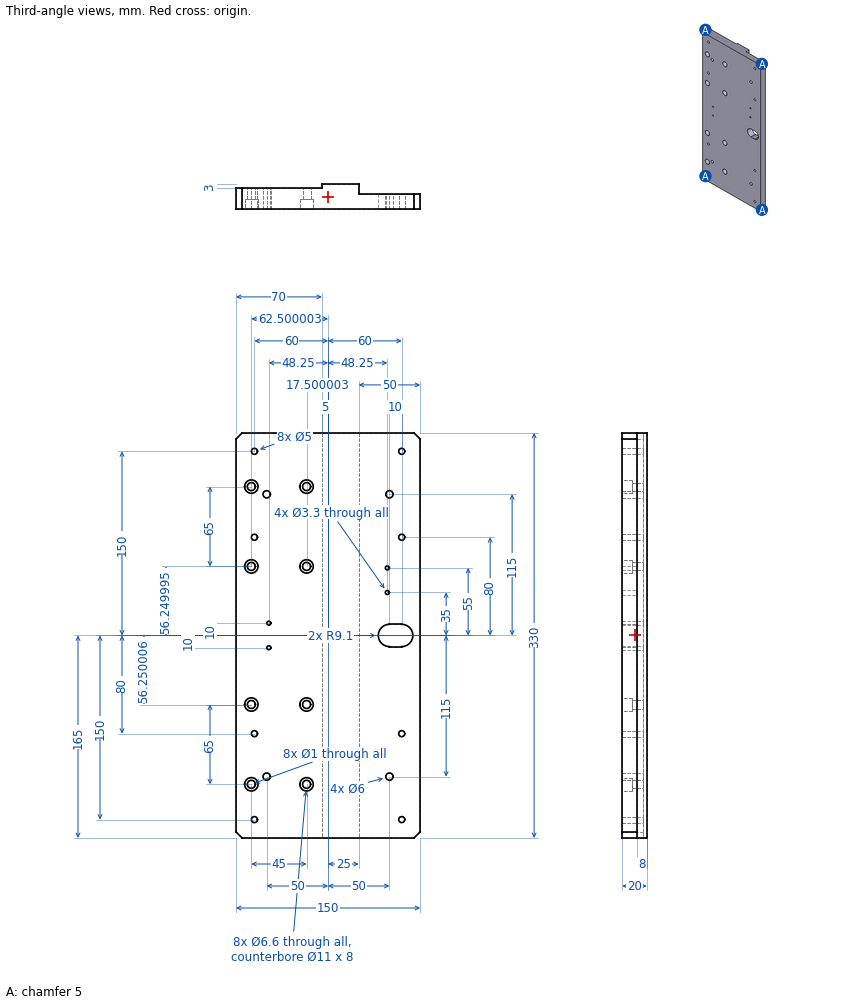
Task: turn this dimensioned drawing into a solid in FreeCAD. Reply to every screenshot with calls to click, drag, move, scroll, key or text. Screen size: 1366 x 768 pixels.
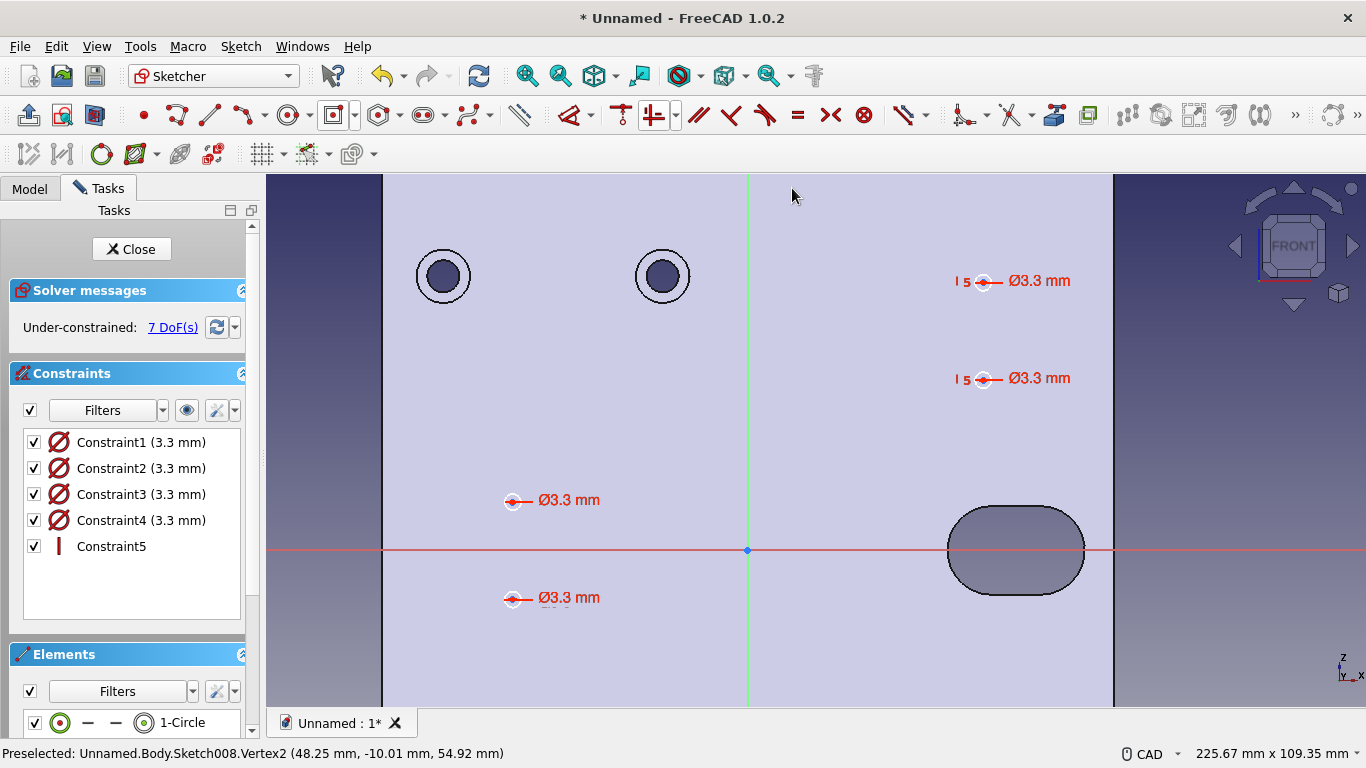
click(513, 502)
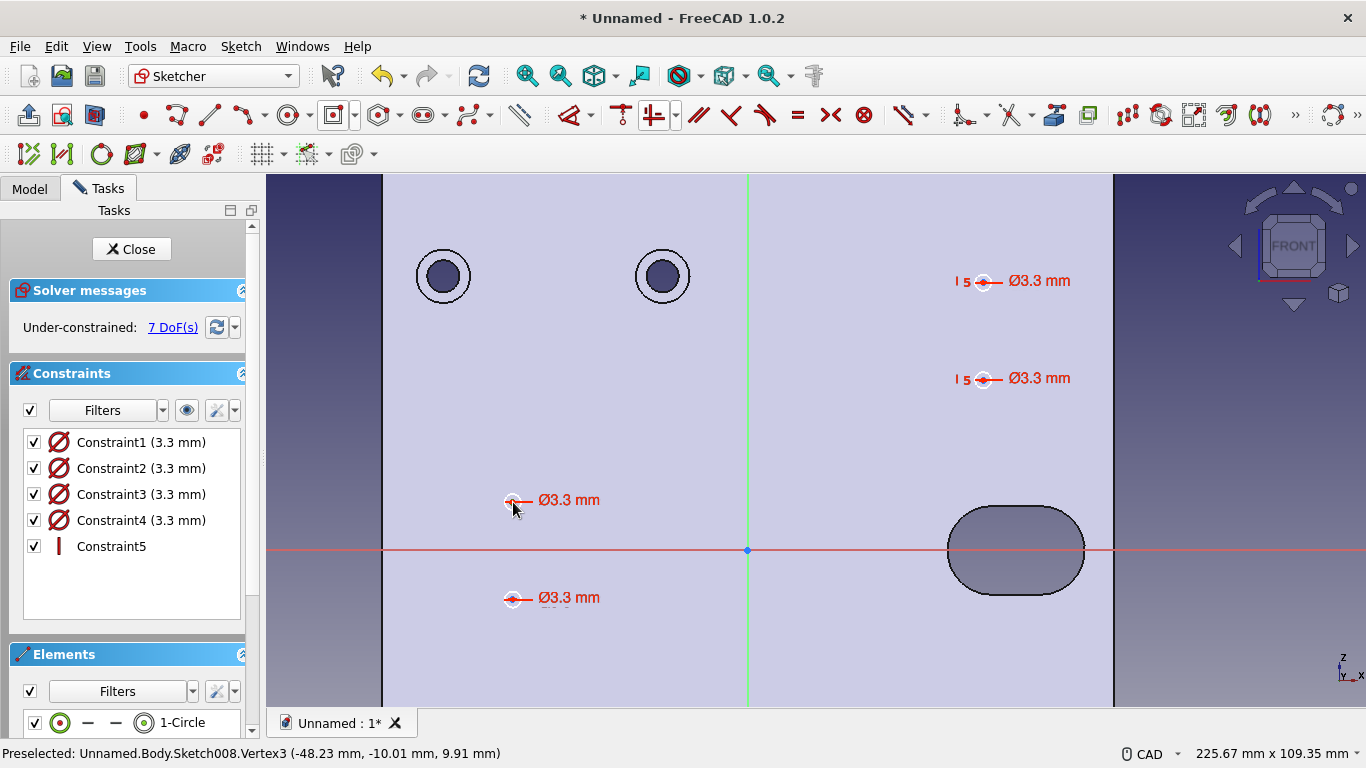
click(513, 600)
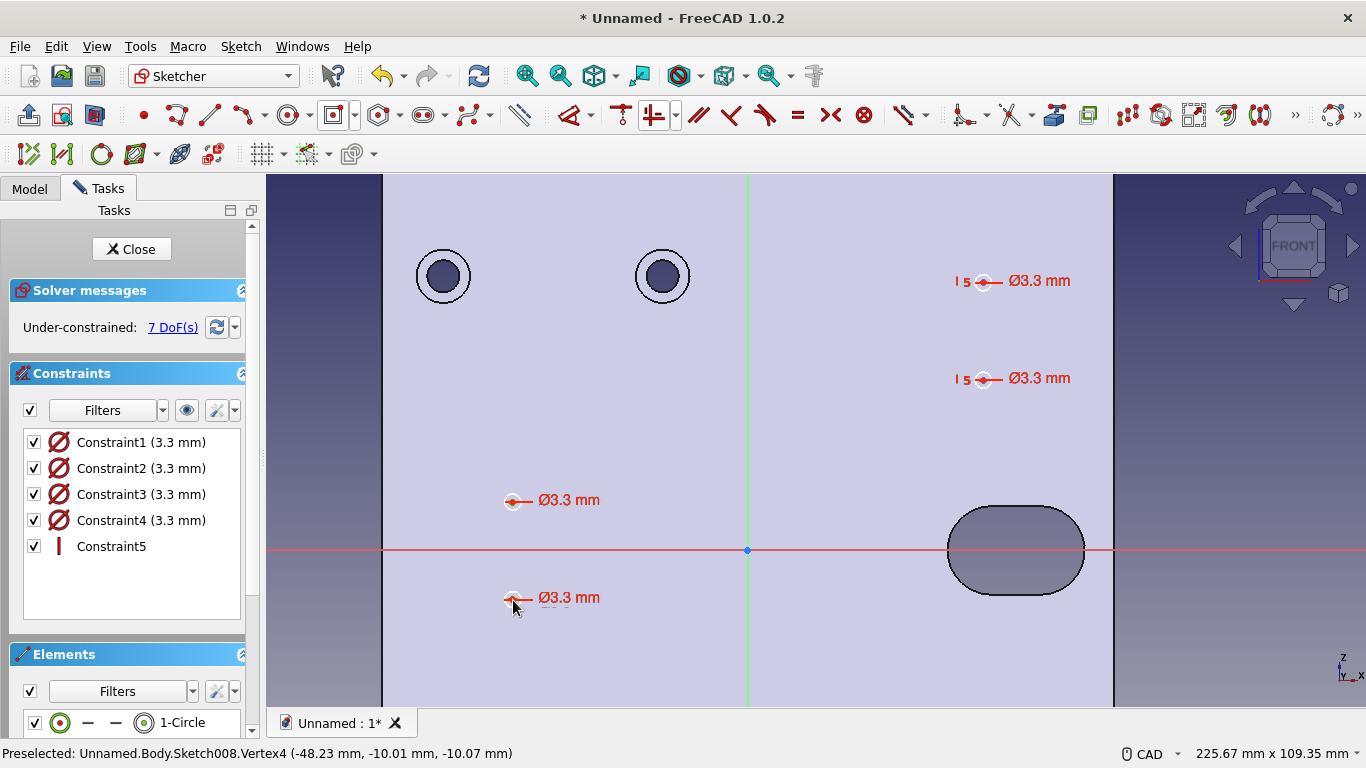
click(676, 116)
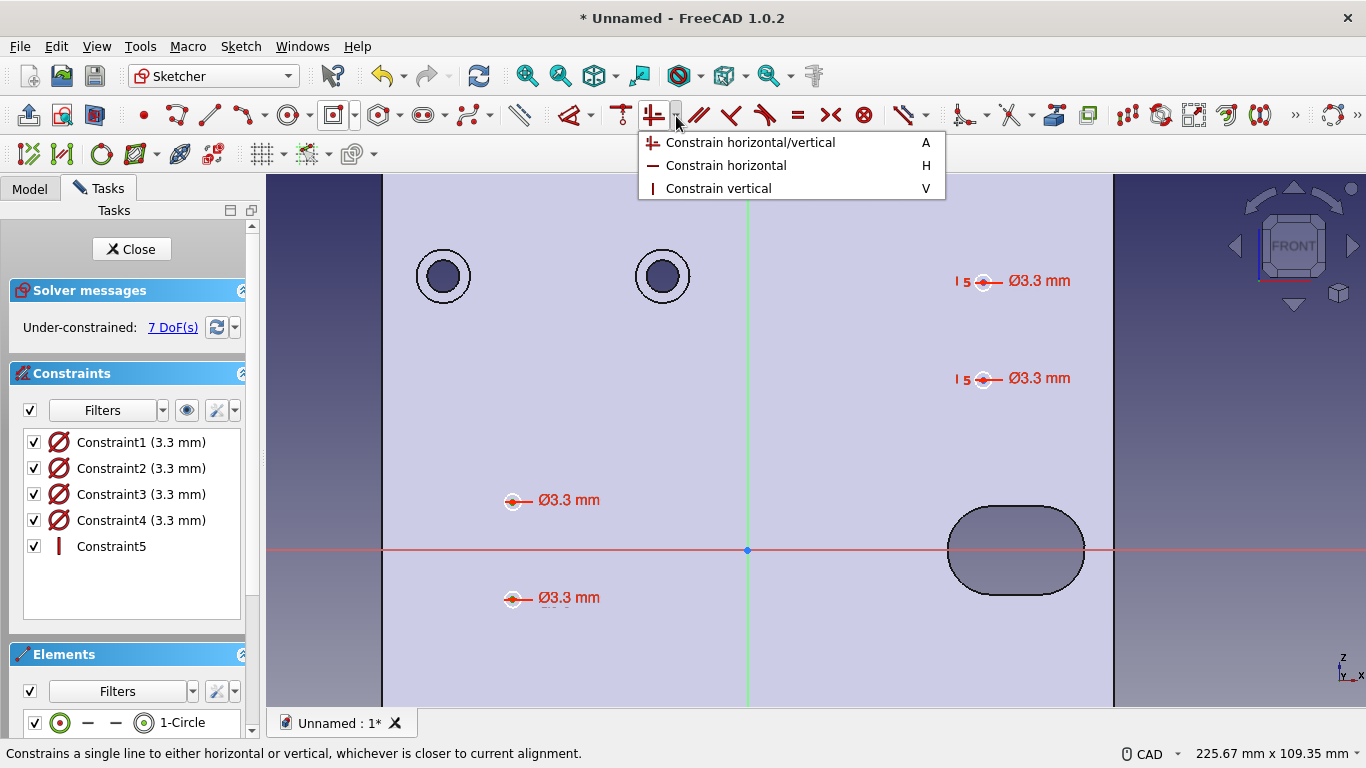
click(792, 188)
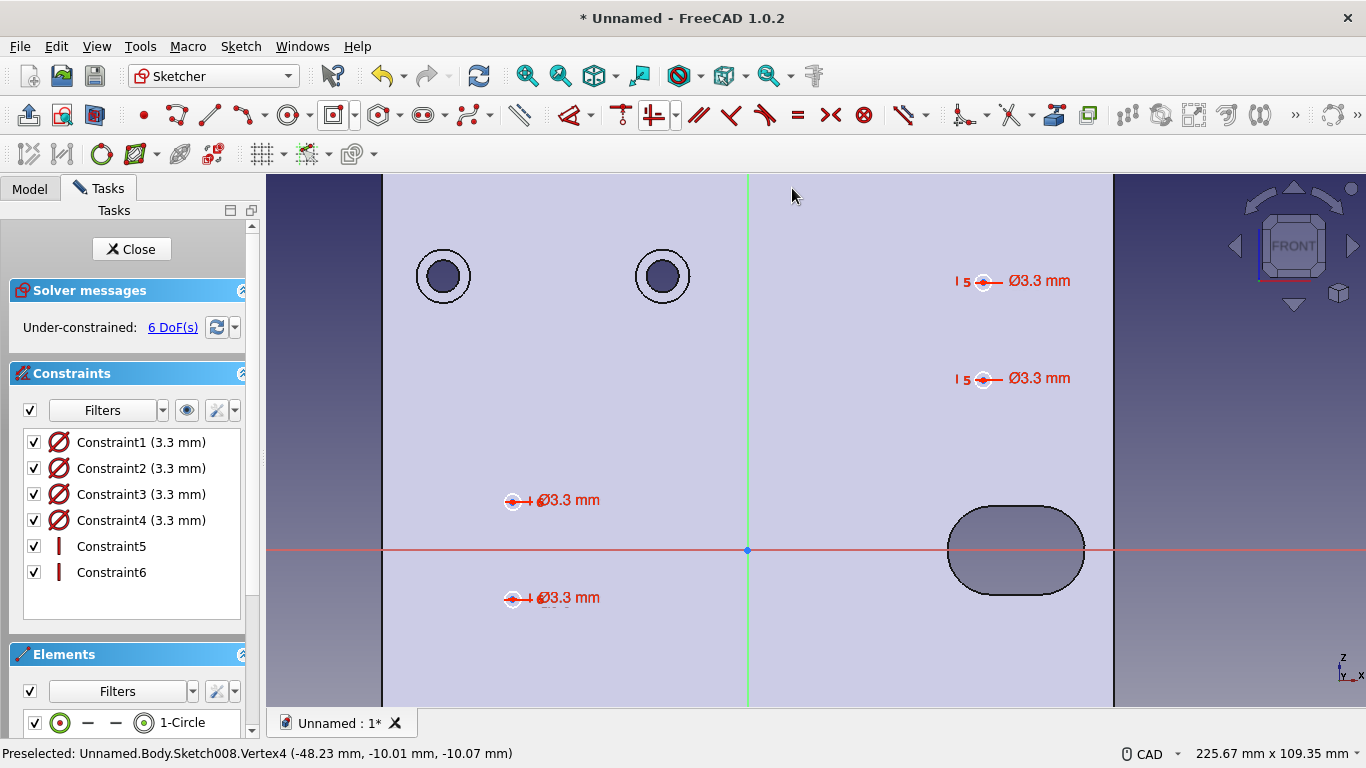
click(568, 116)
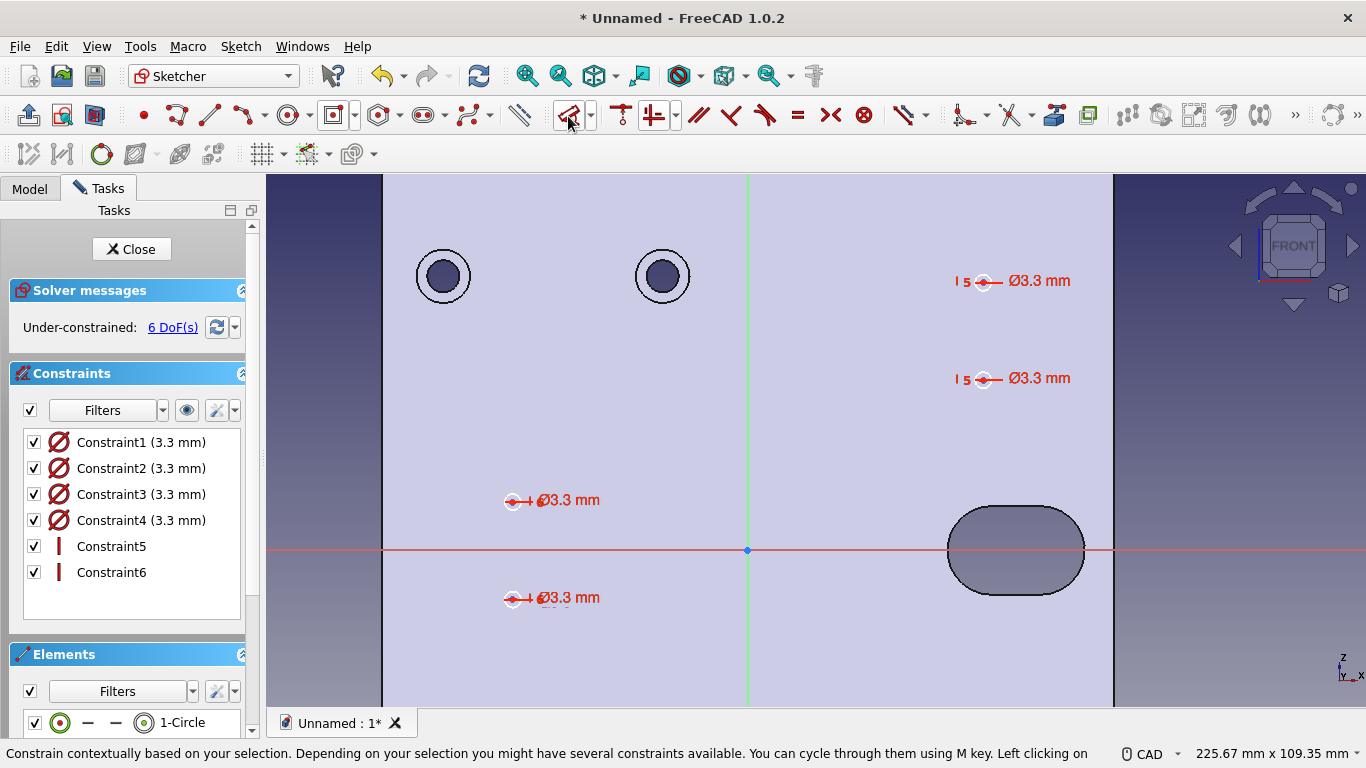
click(983, 380)
click(1017, 465)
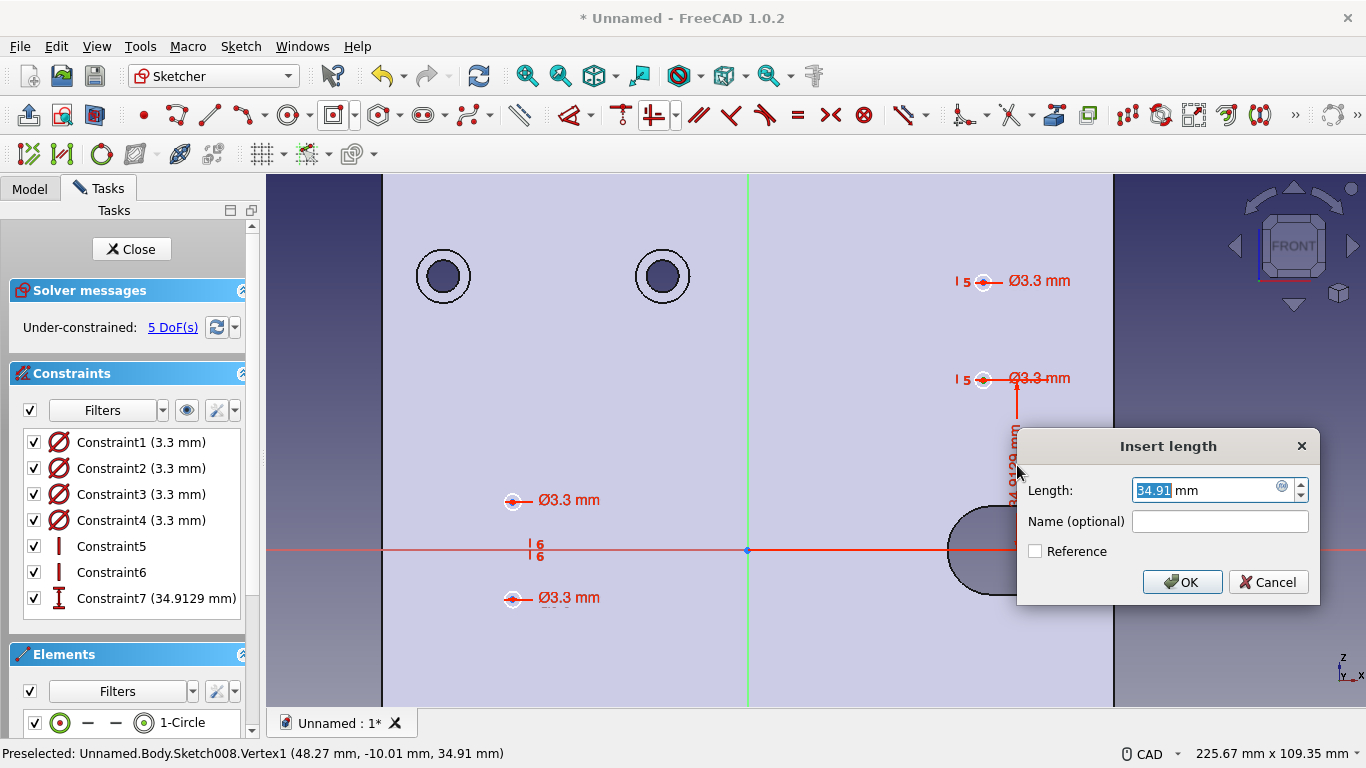
text(35)
key(Return)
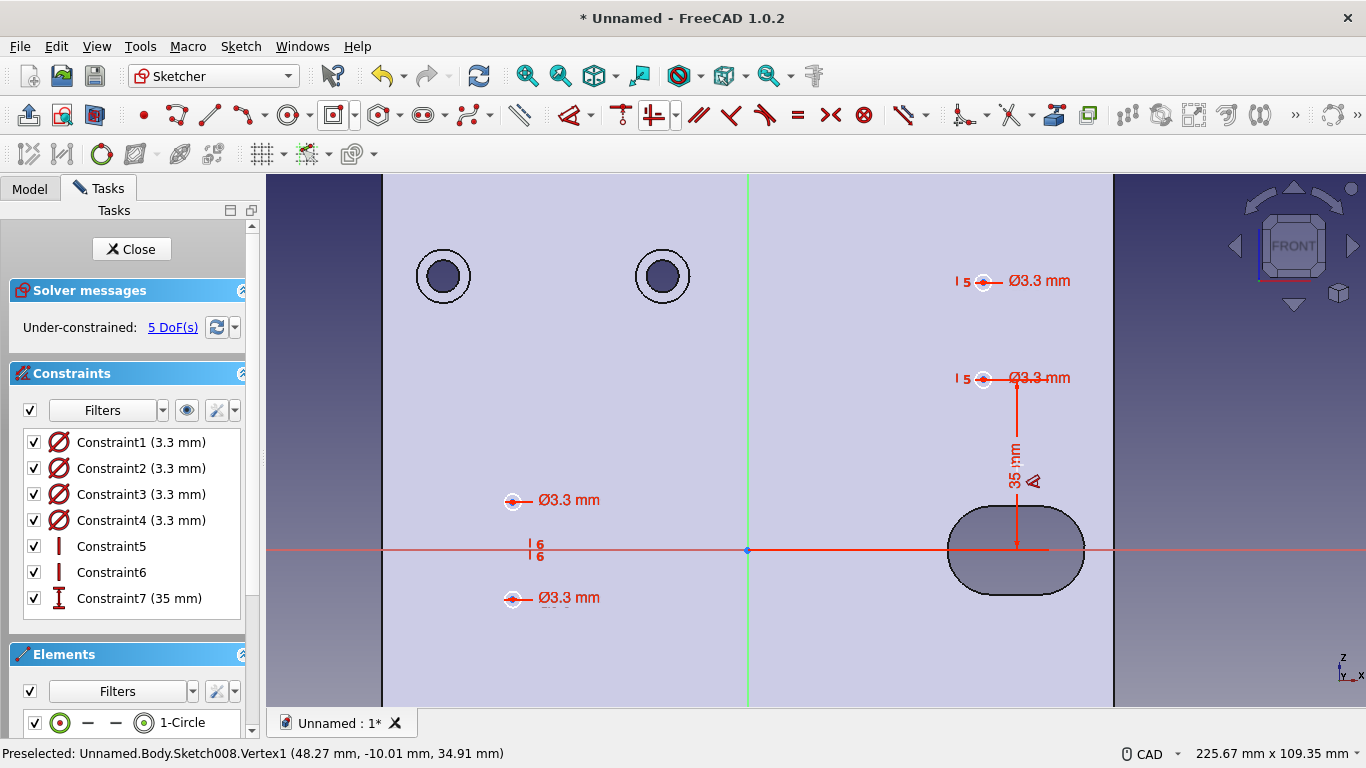
click(983, 283)
click(1017, 417)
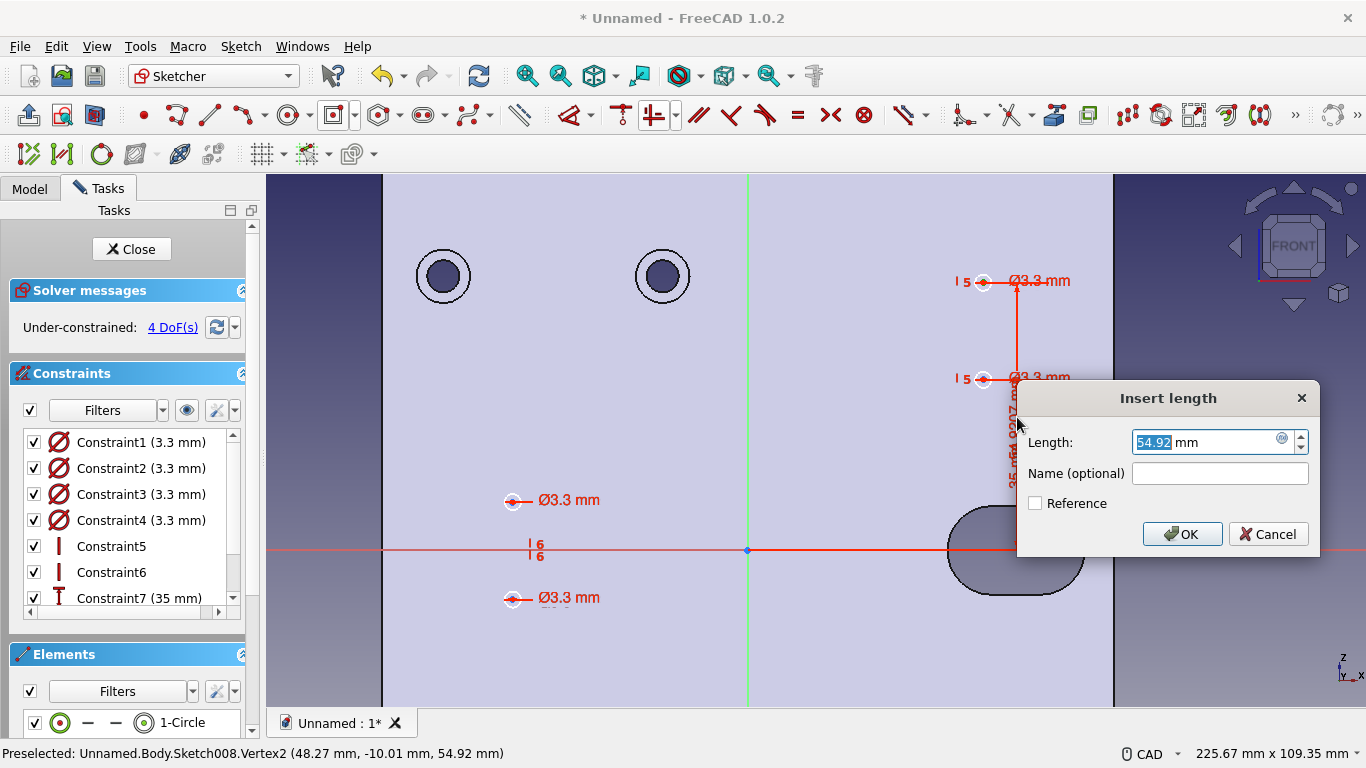
text(55)
key(Return)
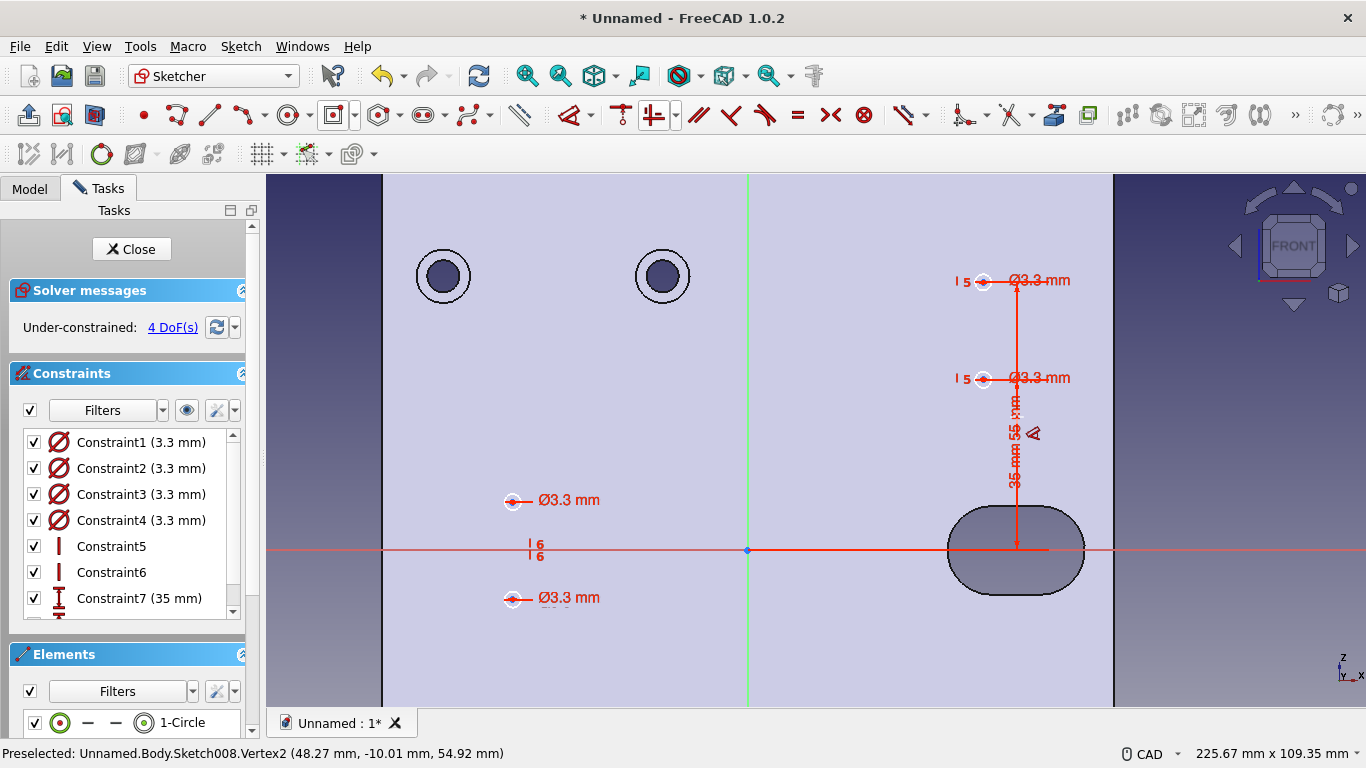
click(513, 502)
click(479, 526)